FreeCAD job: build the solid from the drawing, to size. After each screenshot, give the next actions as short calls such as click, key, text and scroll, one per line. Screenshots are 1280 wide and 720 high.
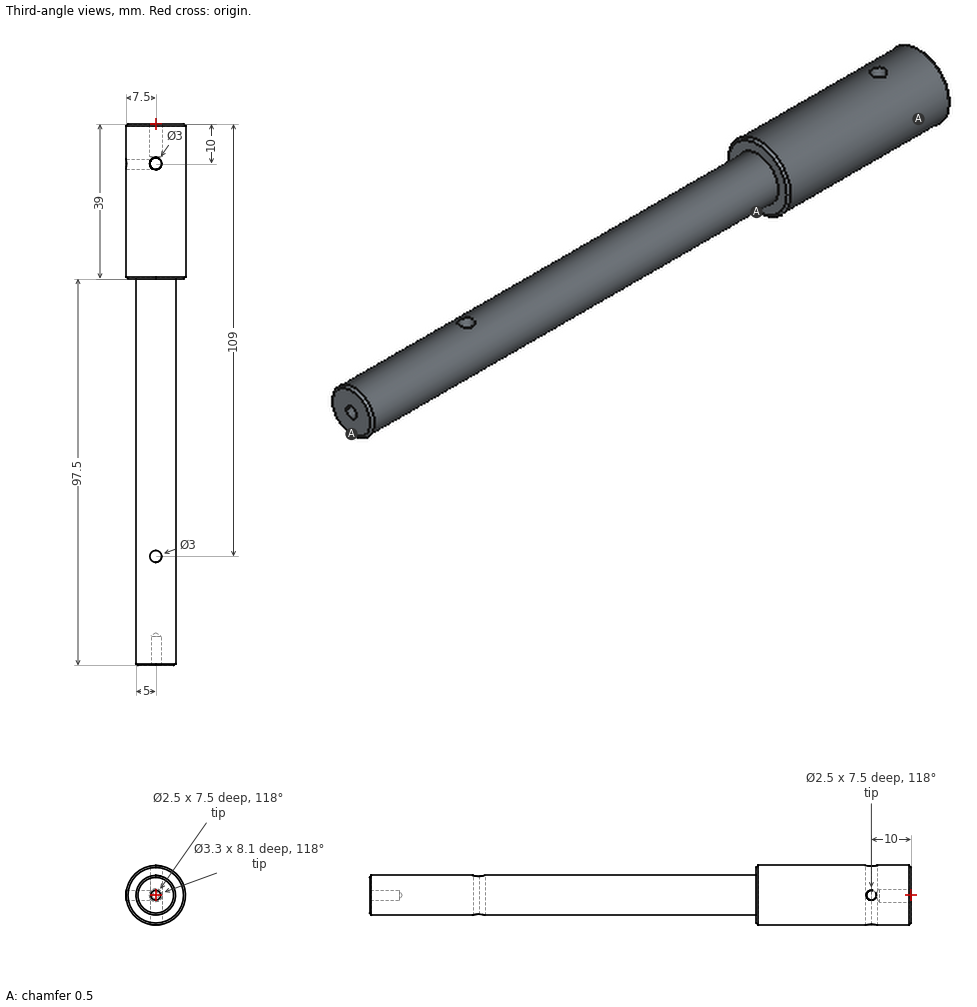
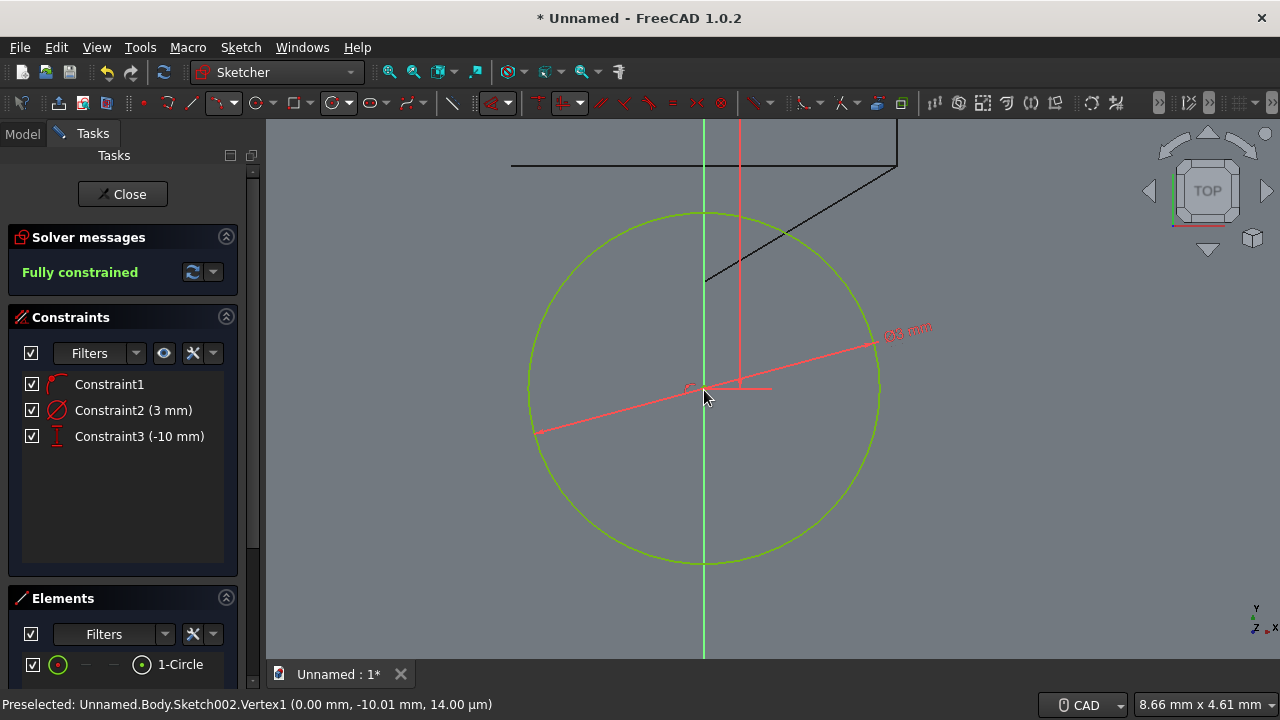
click(123, 194)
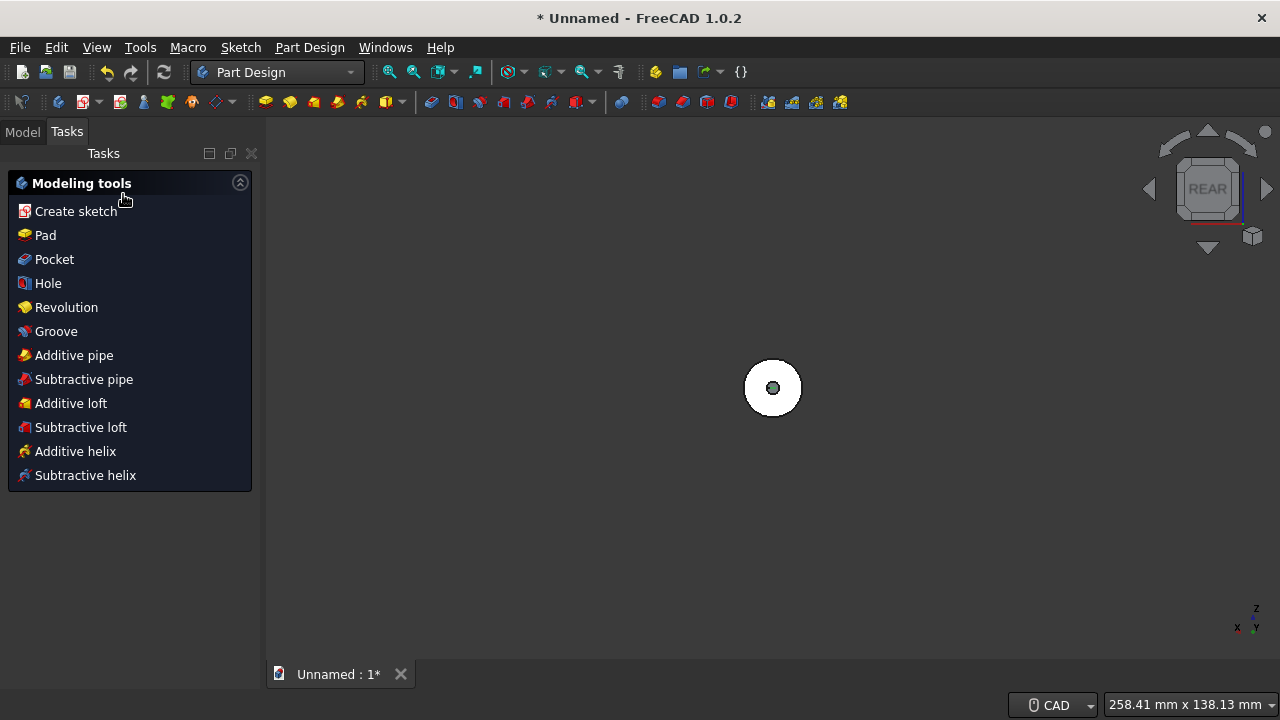
click(432, 102)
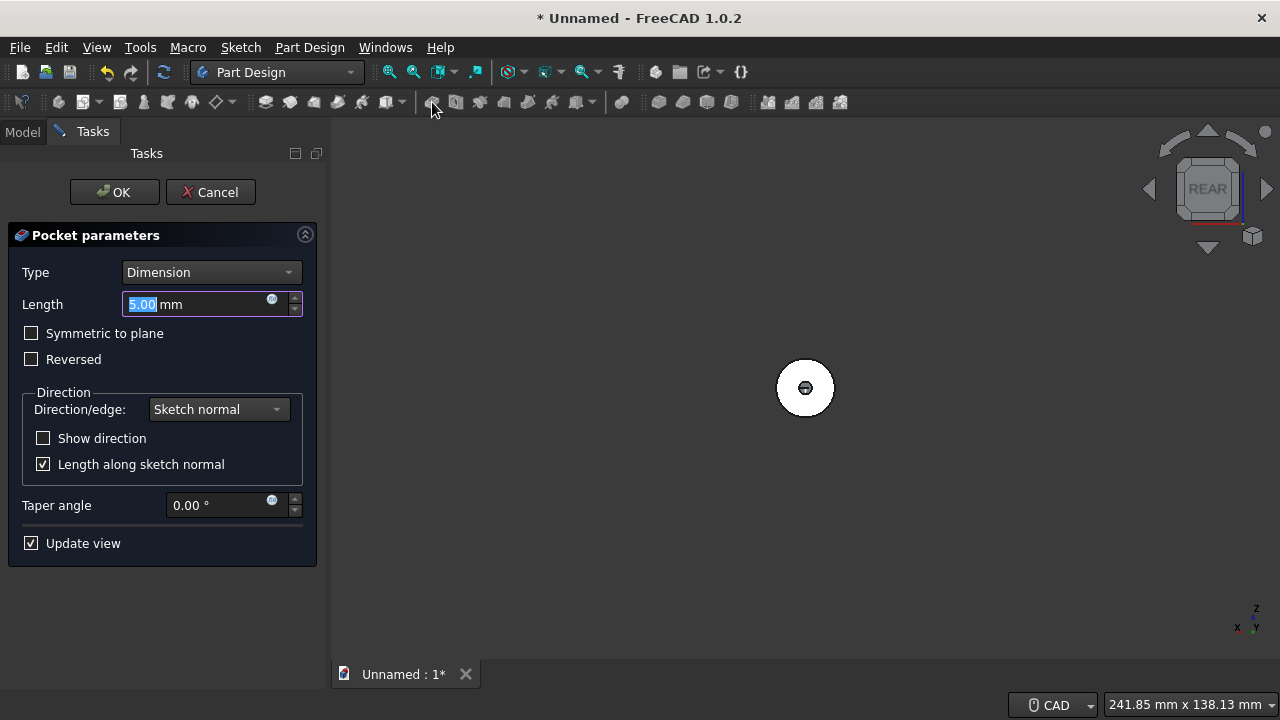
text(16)
key(Tab)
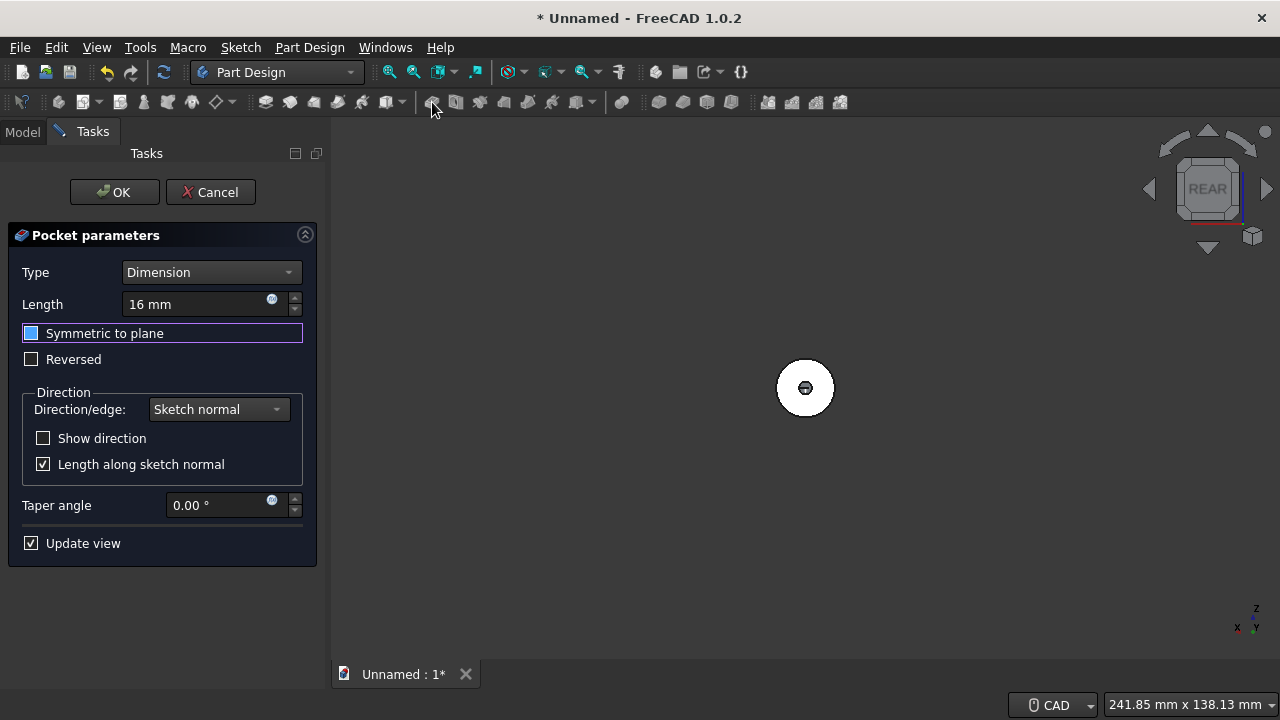
click(30, 333)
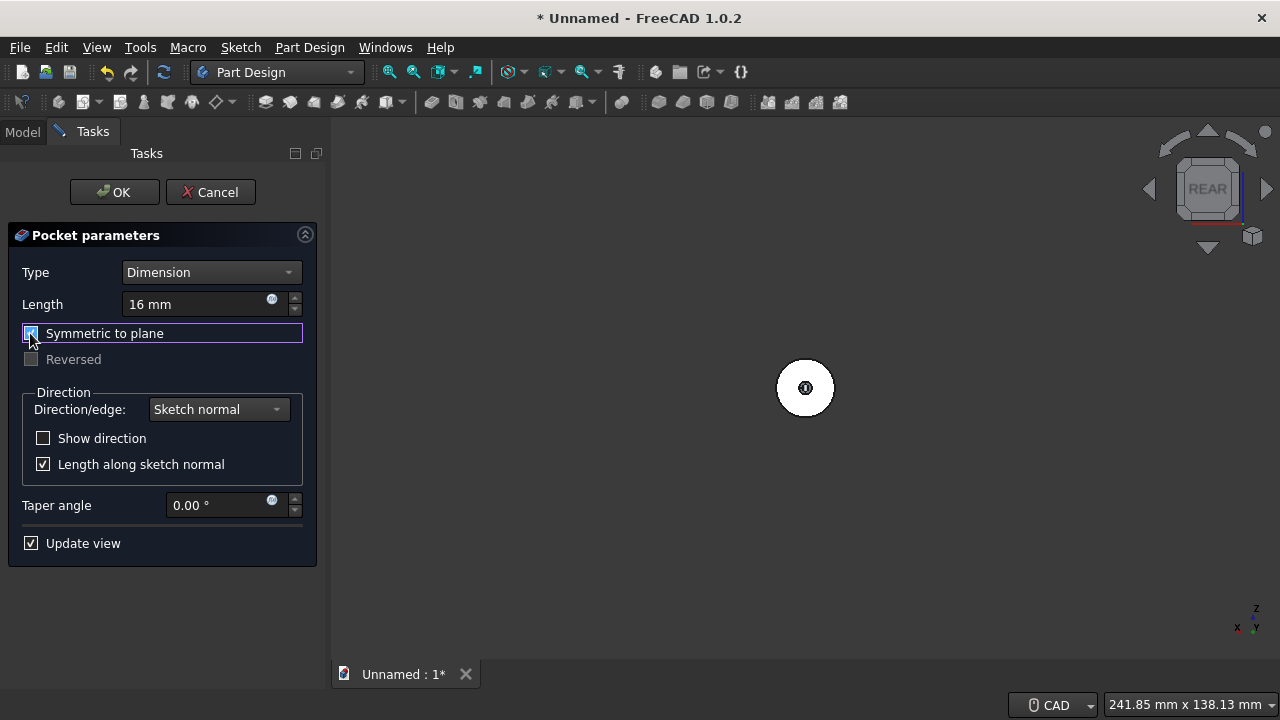
click(115, 192)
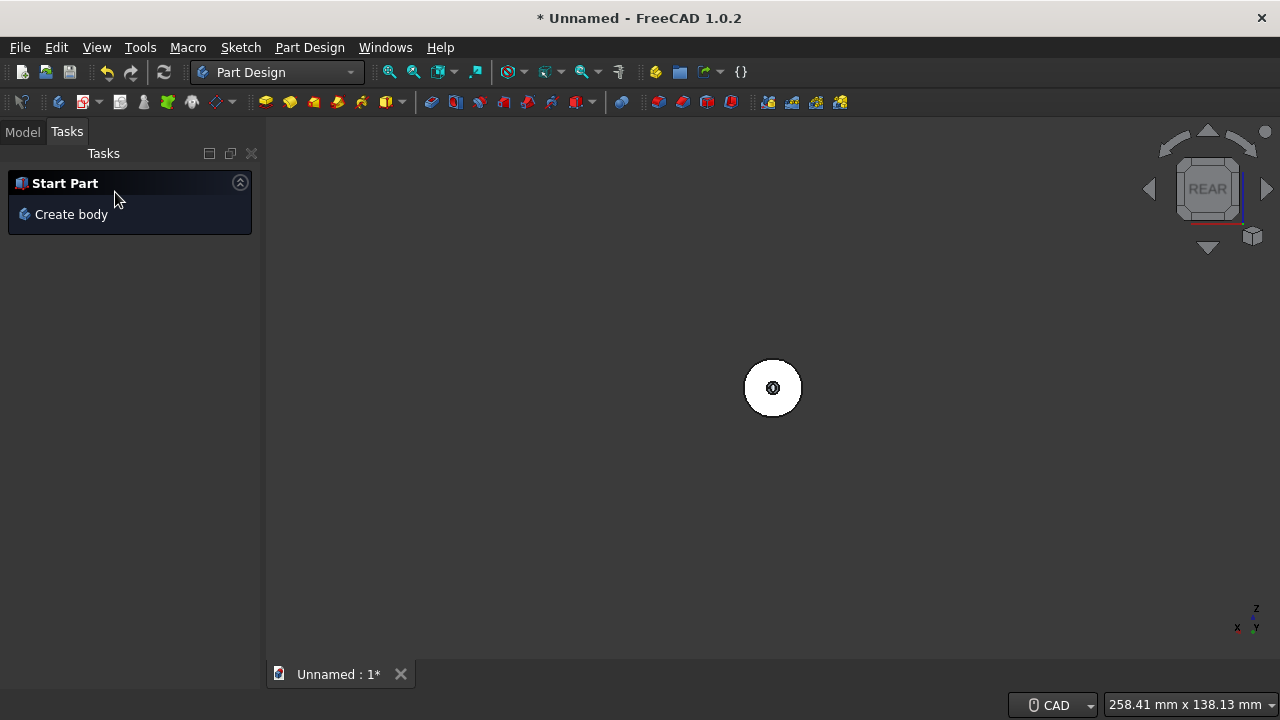
click(390, 72)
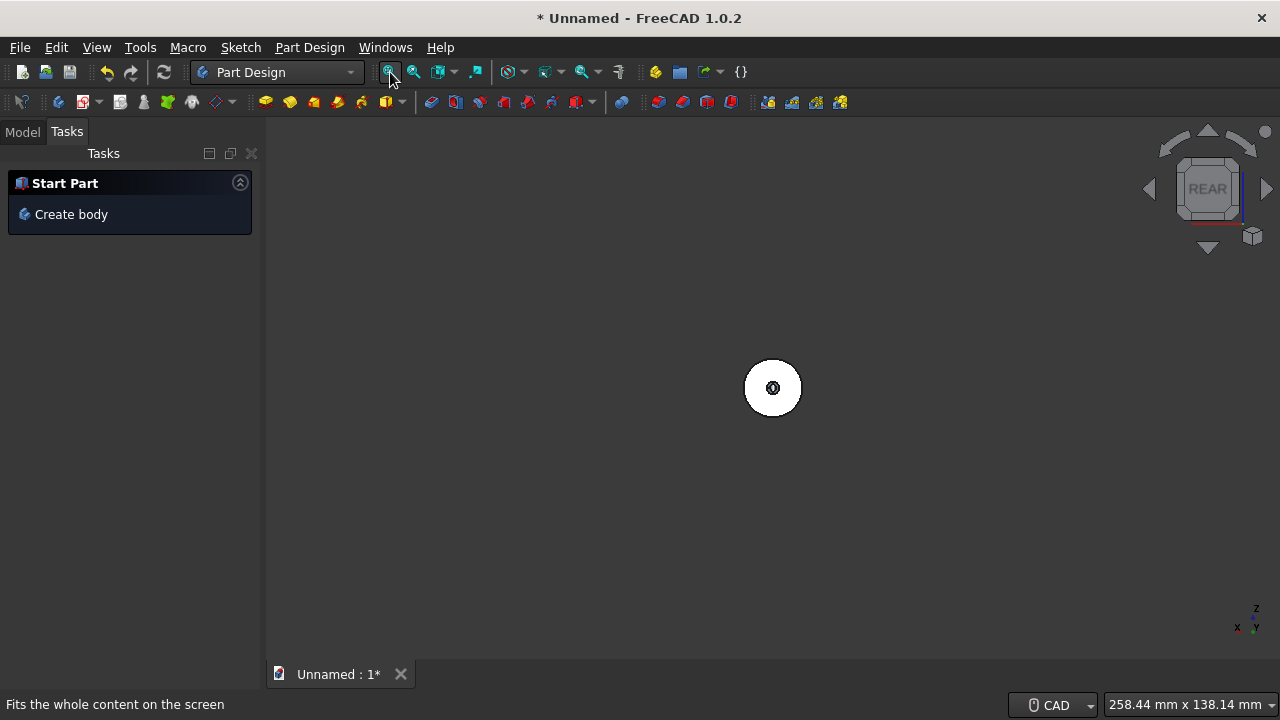
key(0)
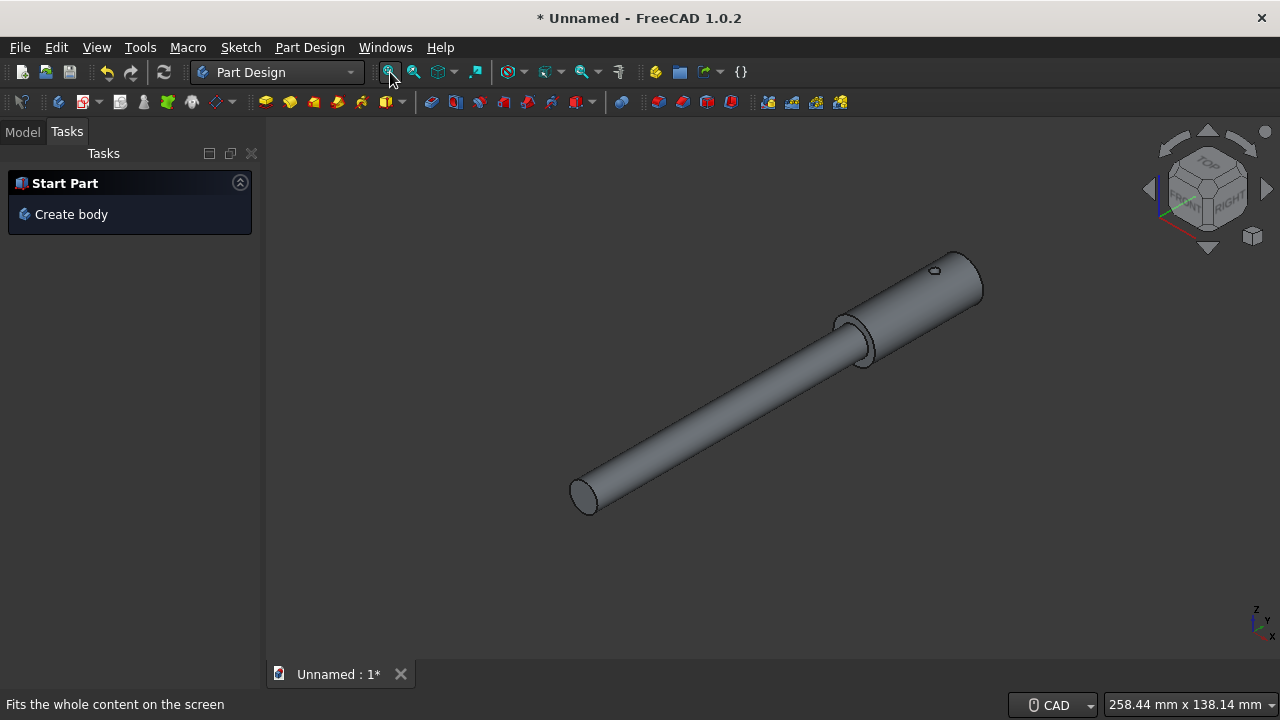
click(584, 496)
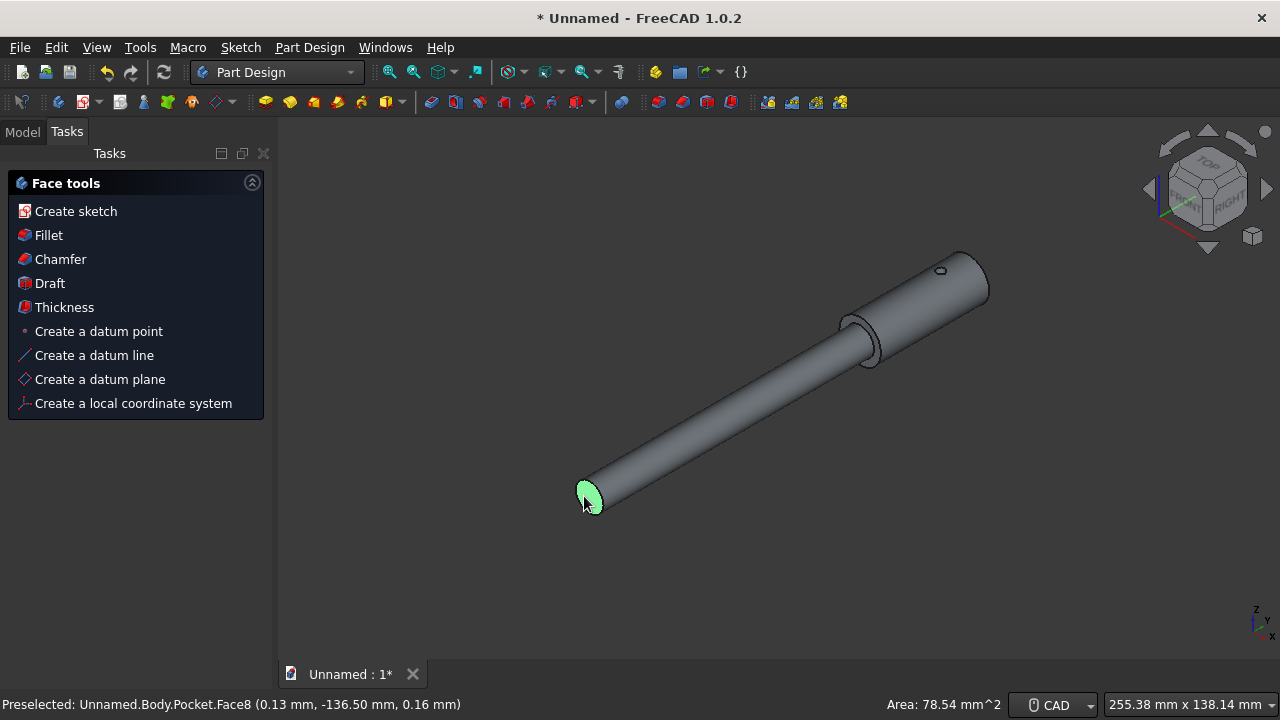
click(84, 102)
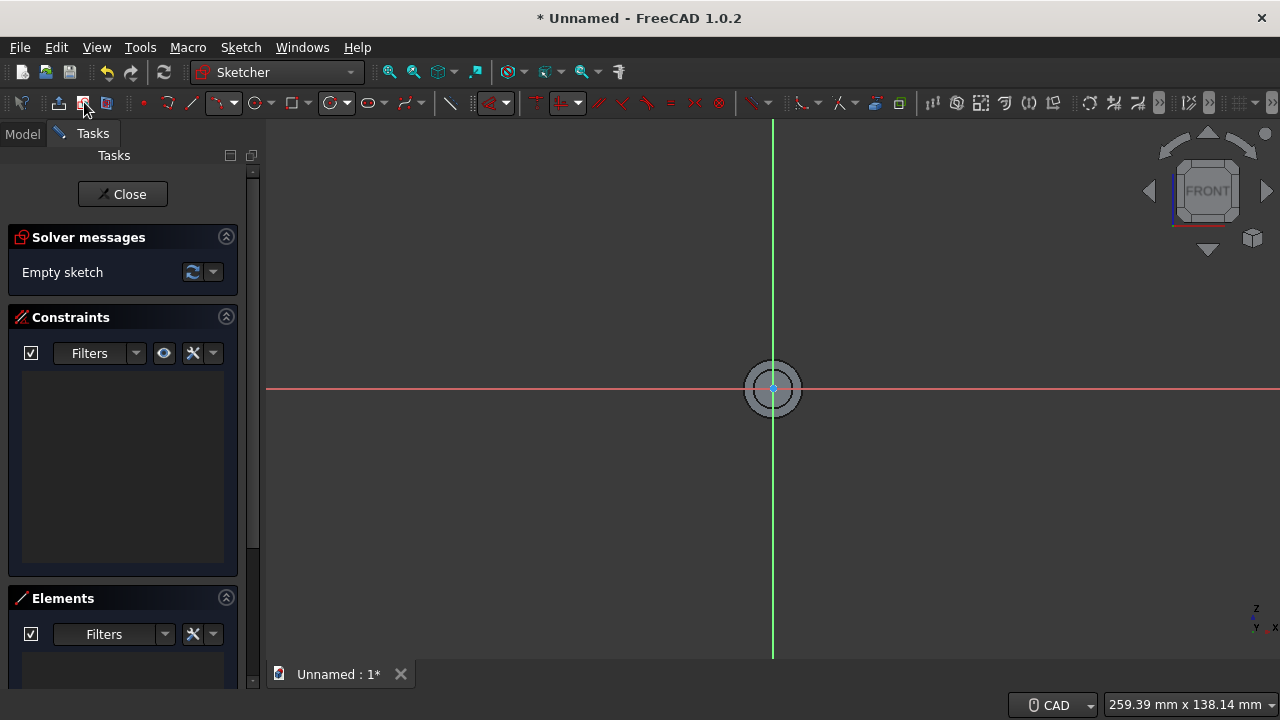
scroll(777, 389, up, 15)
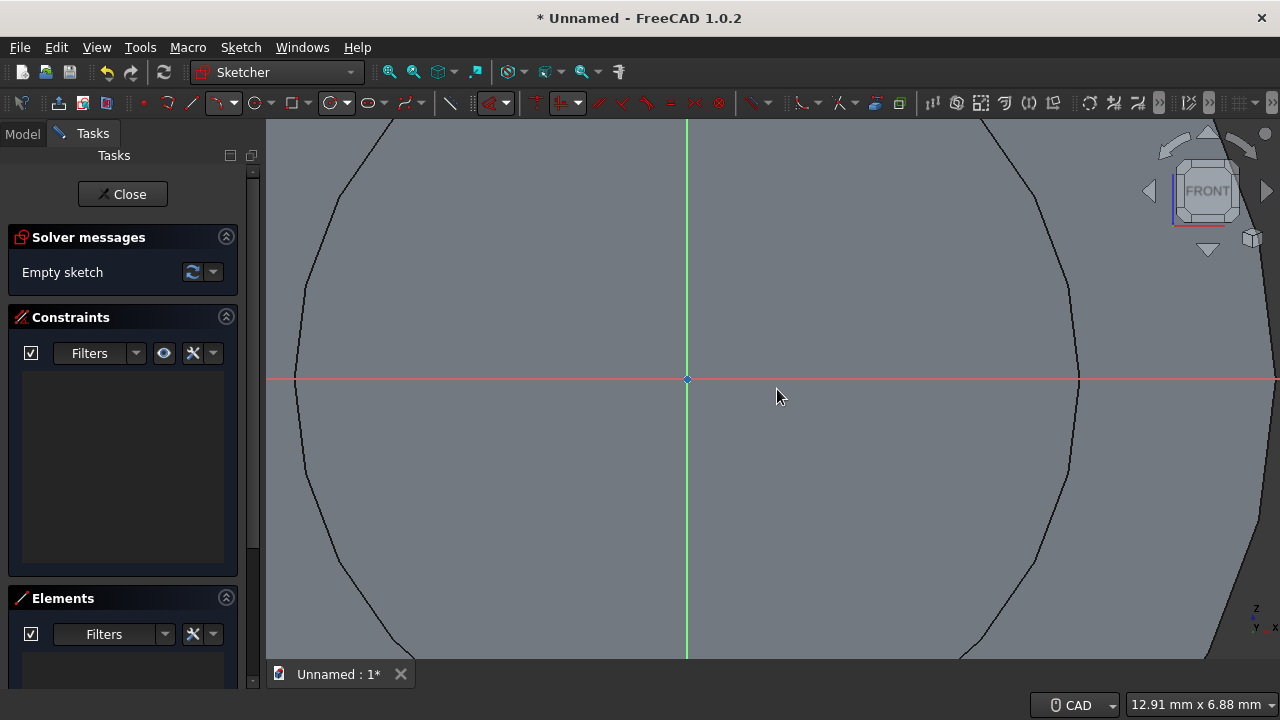
scroll(666, 368, up, 3)